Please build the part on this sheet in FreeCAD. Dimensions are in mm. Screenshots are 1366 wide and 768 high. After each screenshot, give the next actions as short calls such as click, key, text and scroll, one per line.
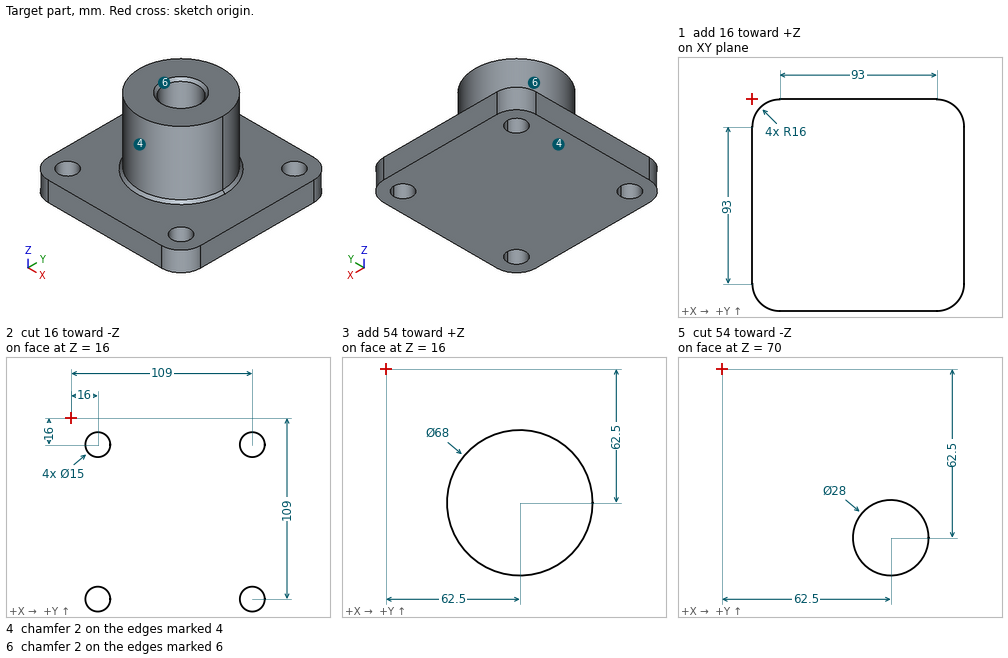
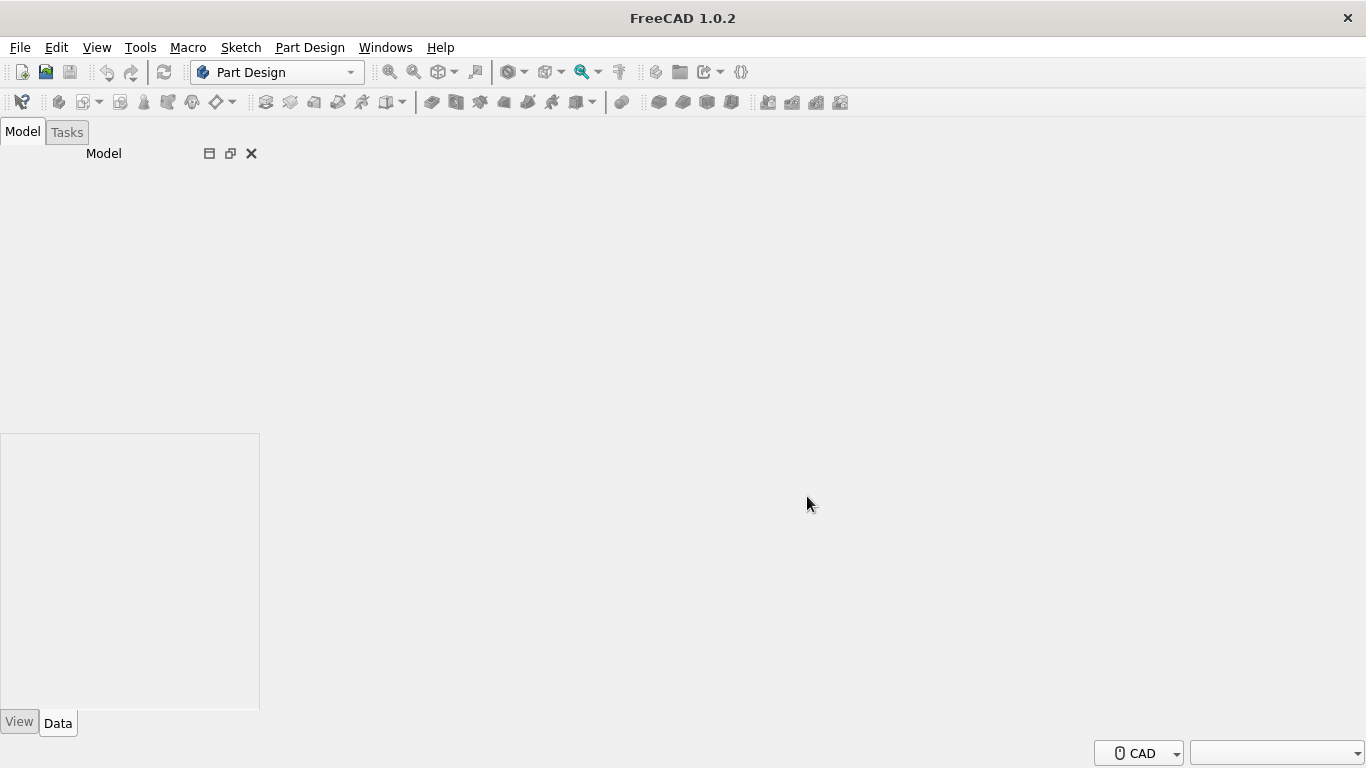
click(22, 72)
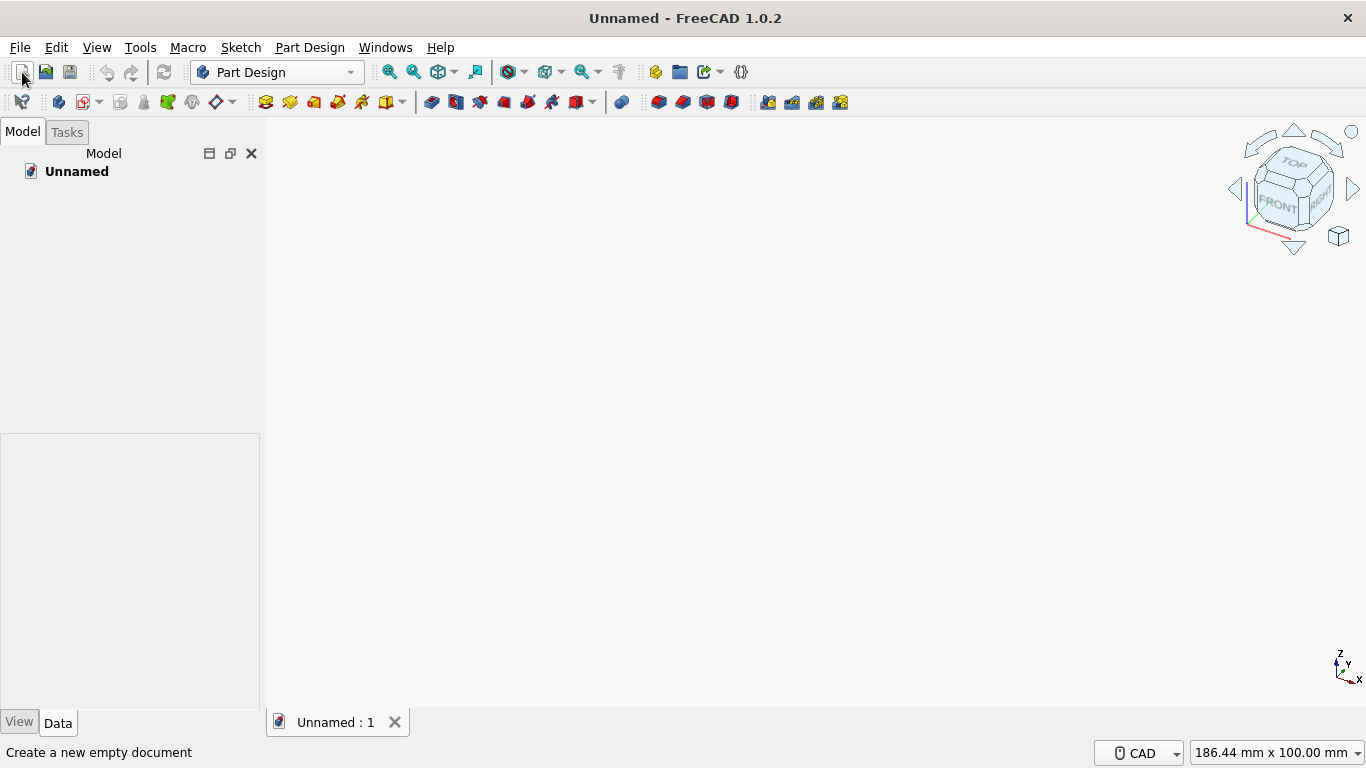
click(84, 102)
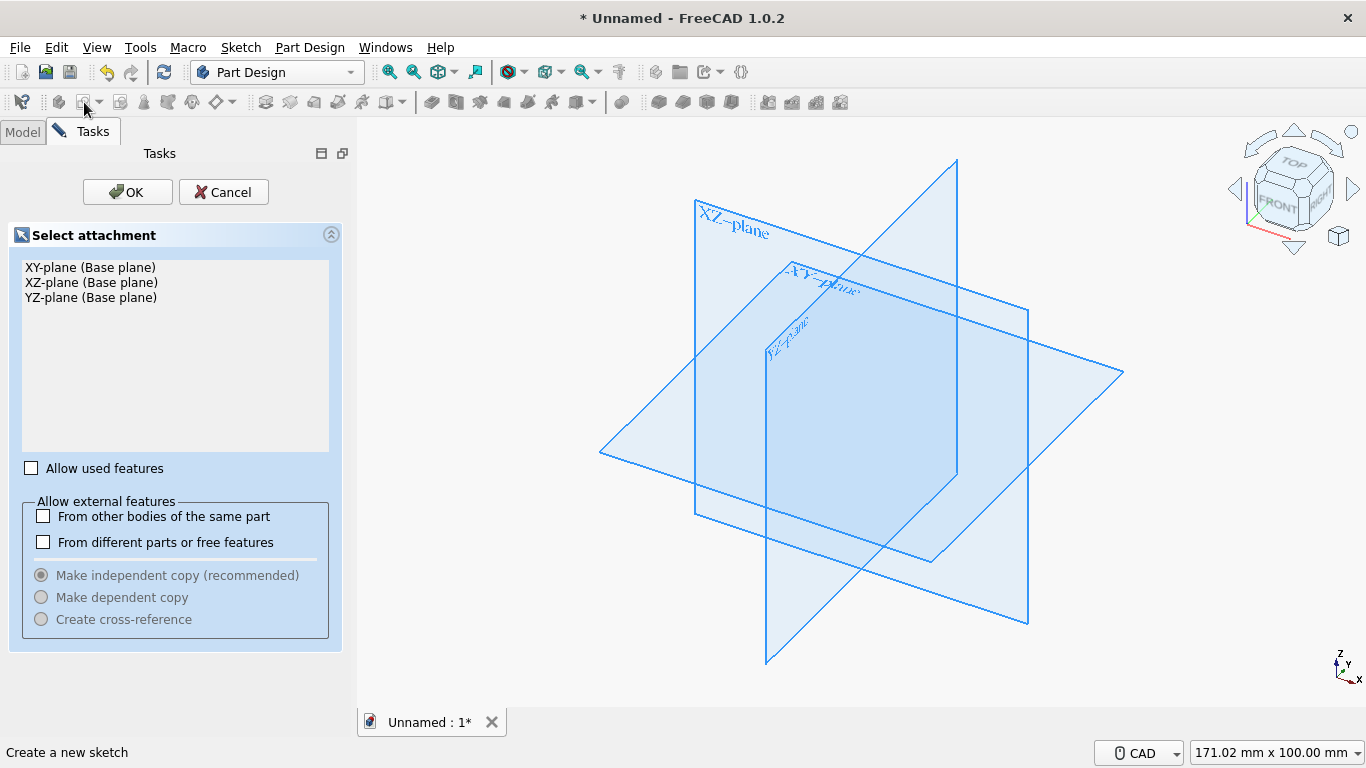
click(82, 268)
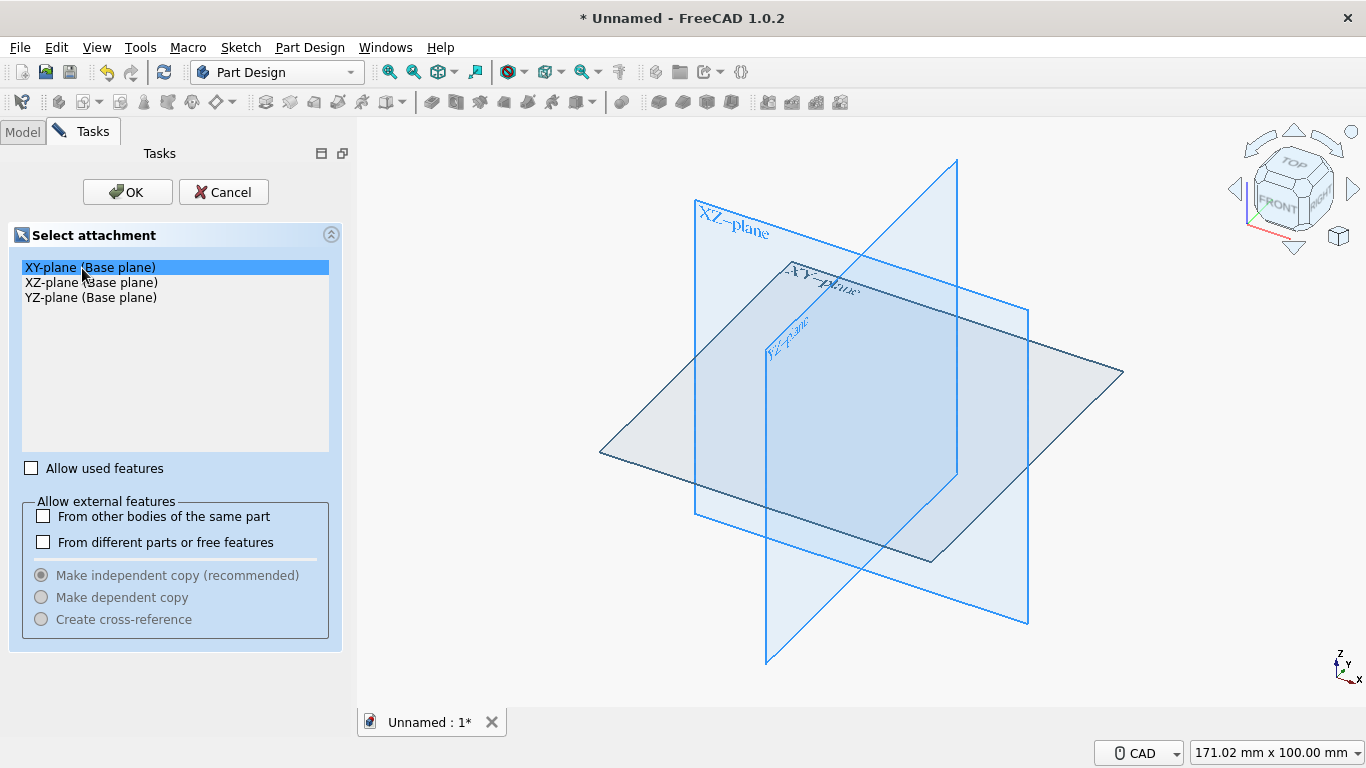
click(128, 192)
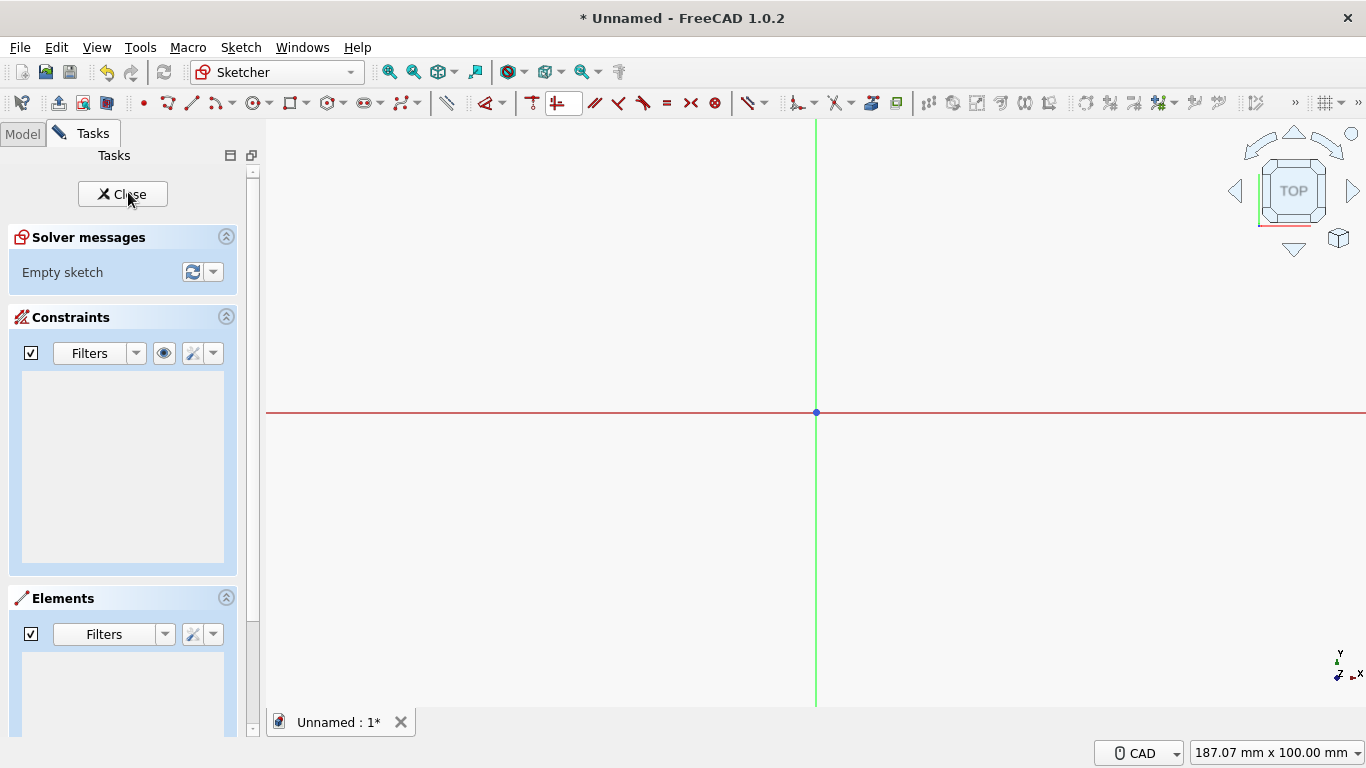
scroll(392, 147, down, 4)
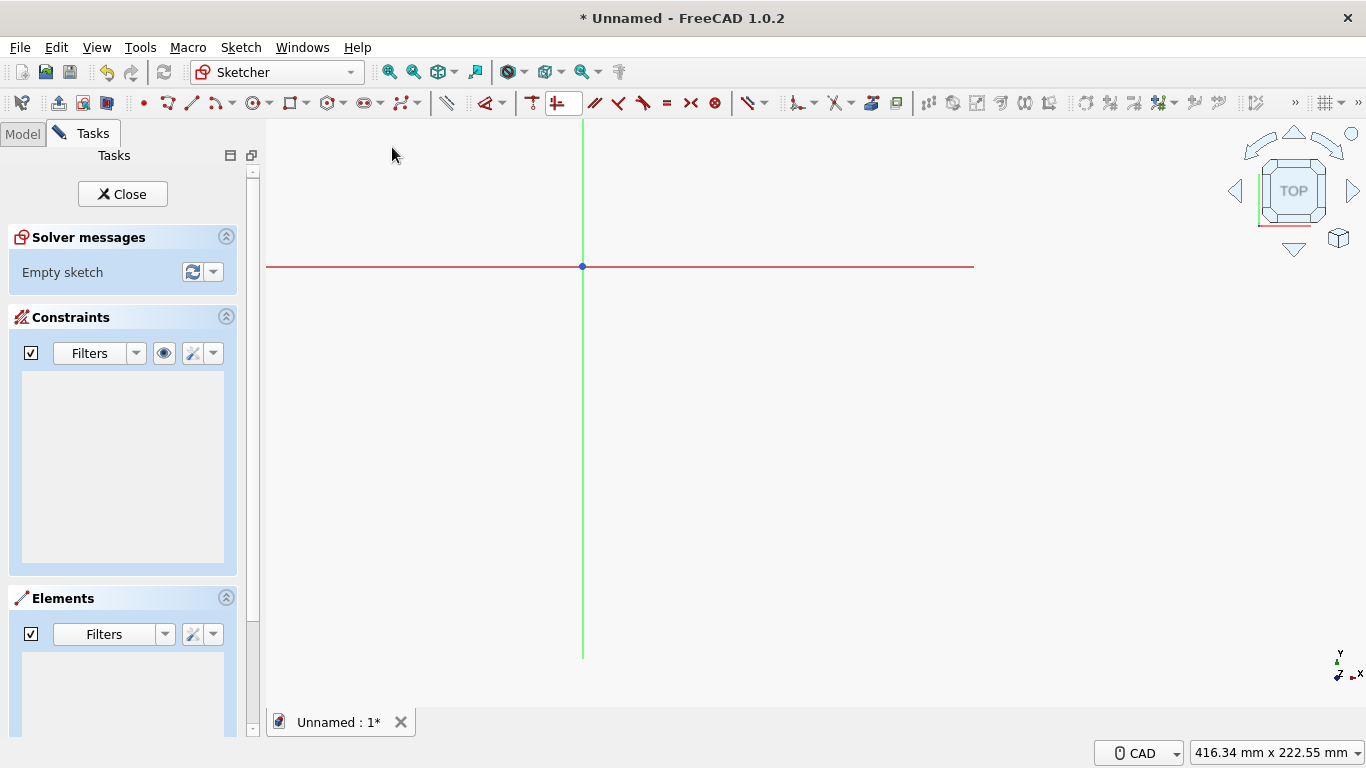
key(g)
key(l)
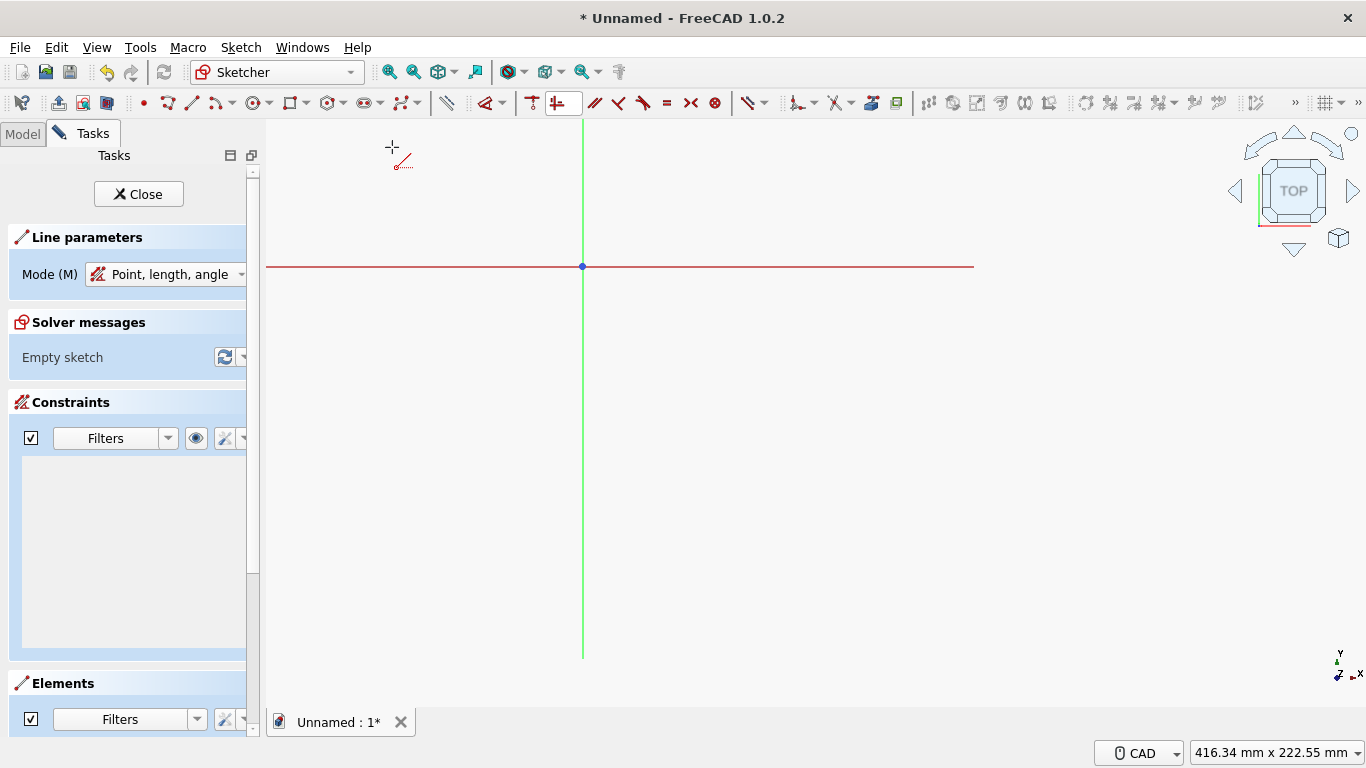
click(871, 267)
click(625, 276)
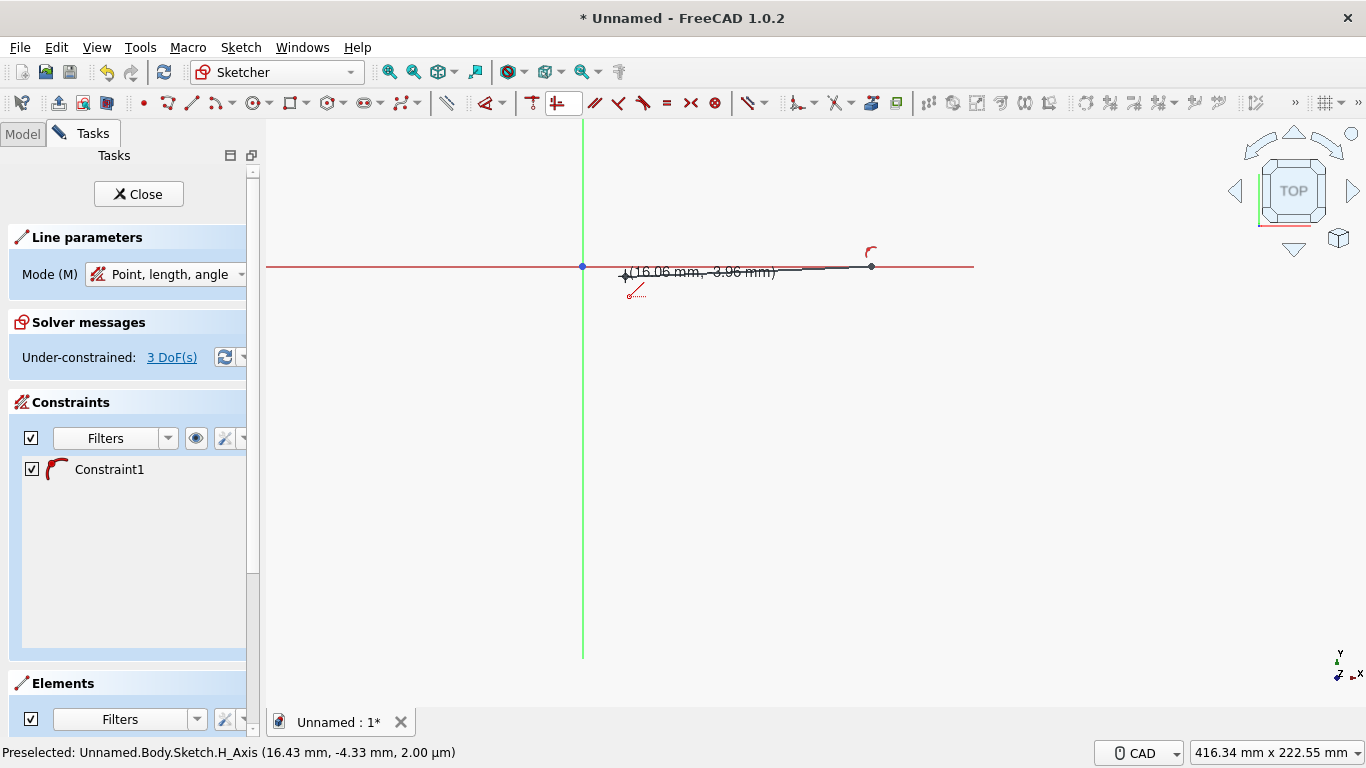
click(583, 309)
click(592, 555)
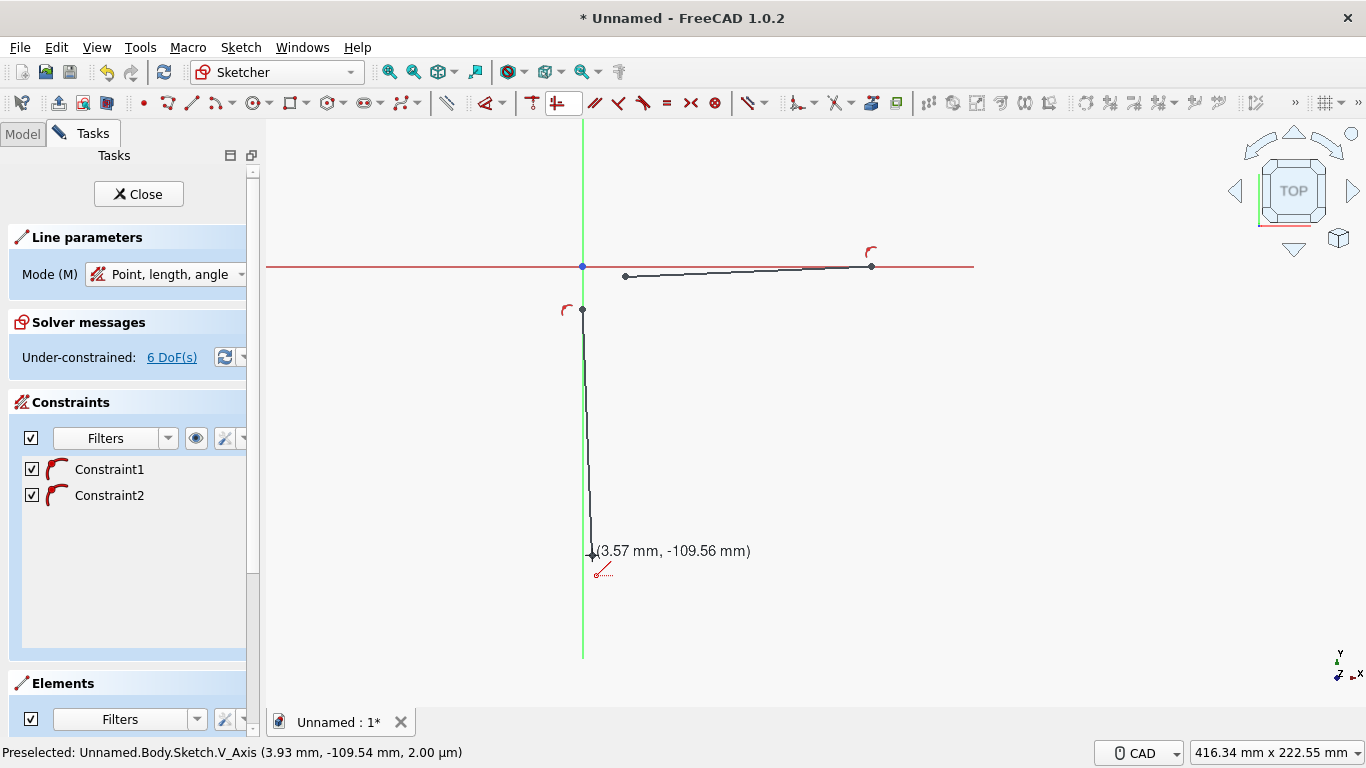
click(625, 597)
click(871, 597)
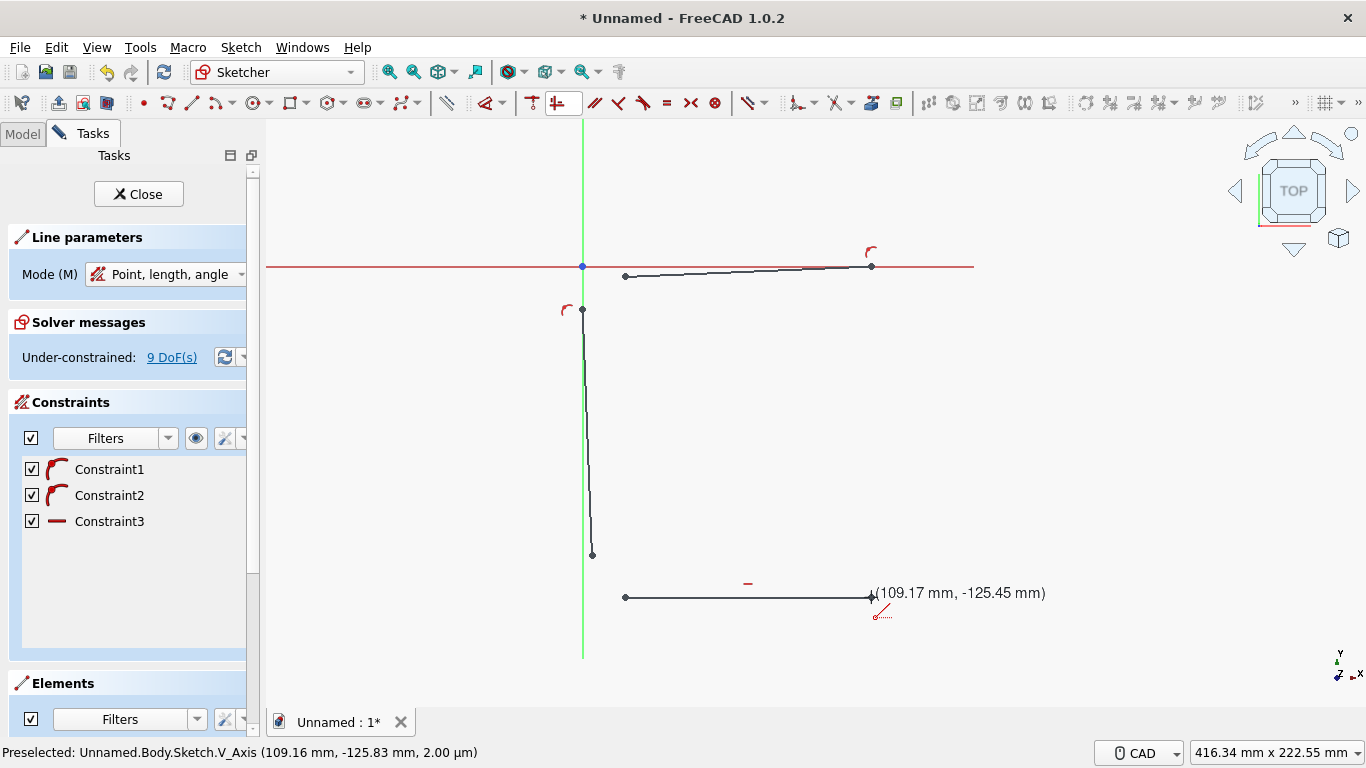
click(913, 555)
click(913, 309)